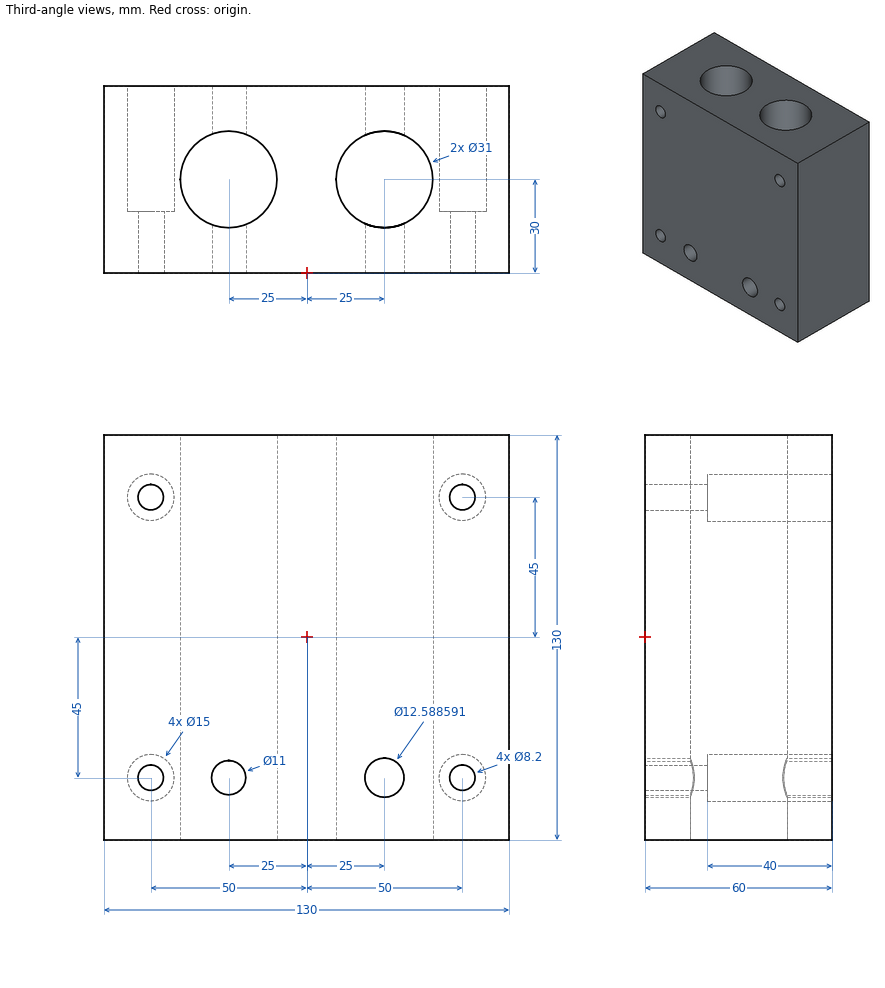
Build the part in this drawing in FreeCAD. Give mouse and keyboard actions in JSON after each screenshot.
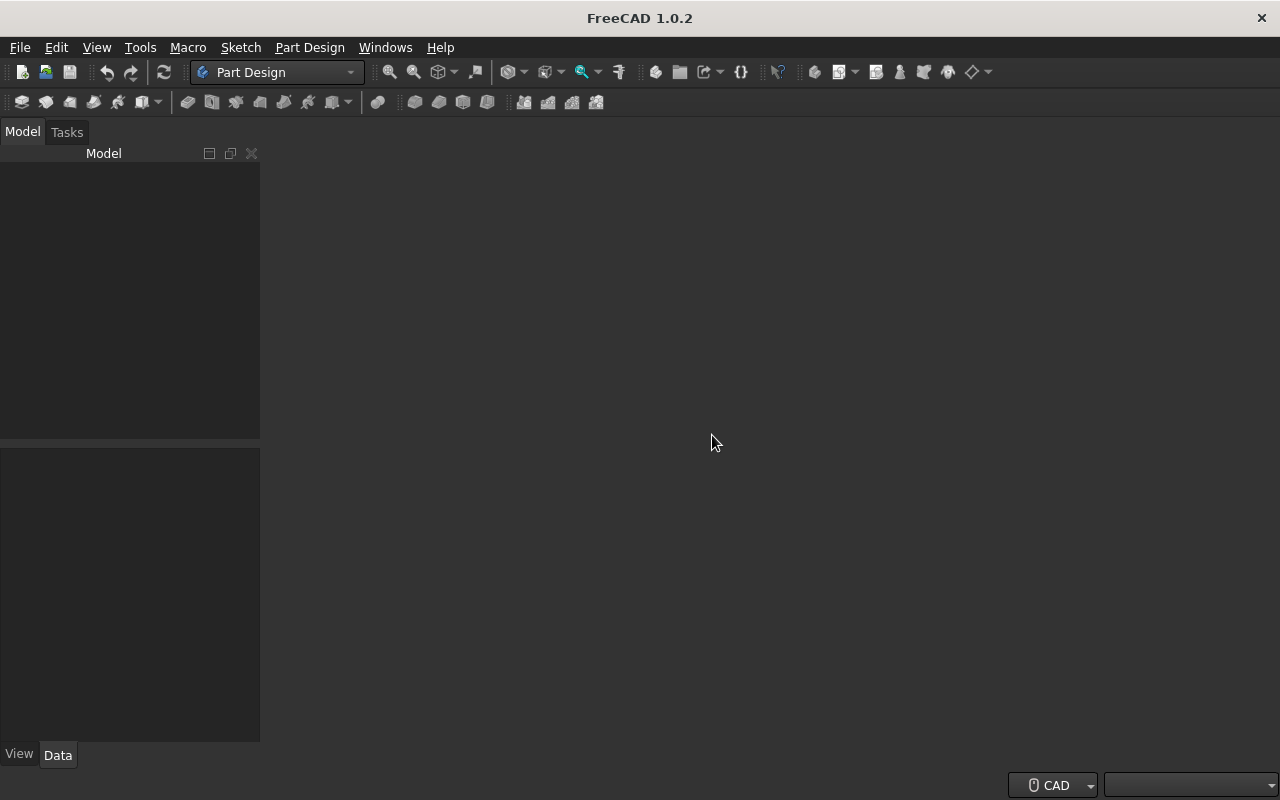
{"action": "key", "text": "ctrl+n"}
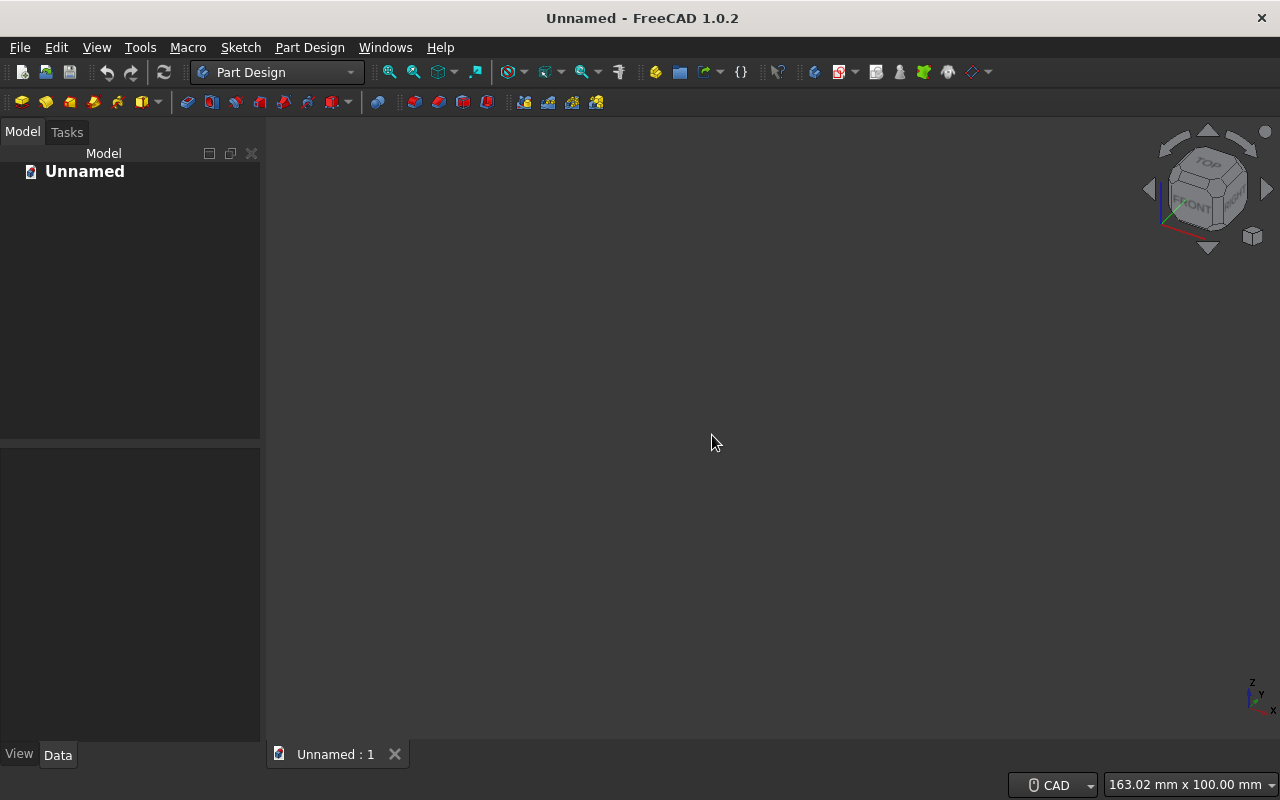
{"action": "left_click", "coordinate": [840, 72]}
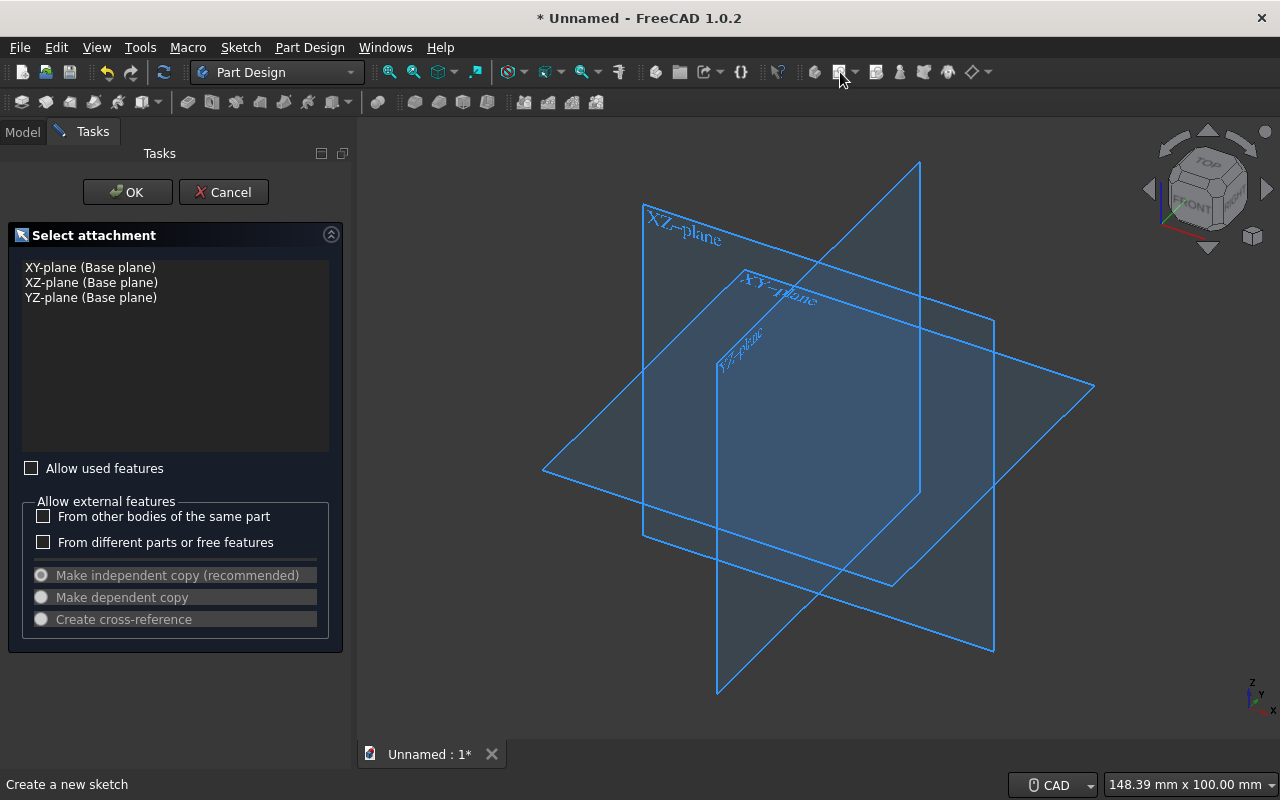
{"action": "left_click", "coordinate": [82, 282]}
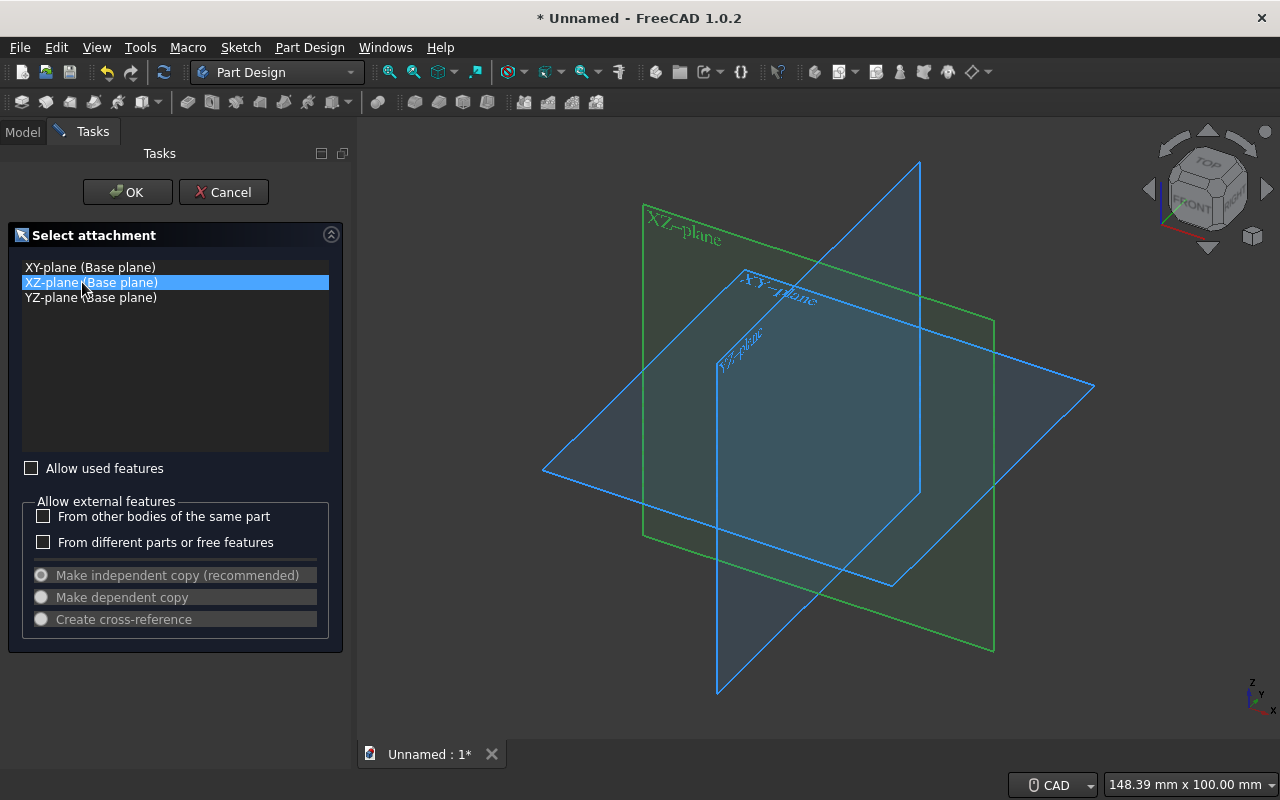
{"action": "left_click", "coordinate": [128, 192]}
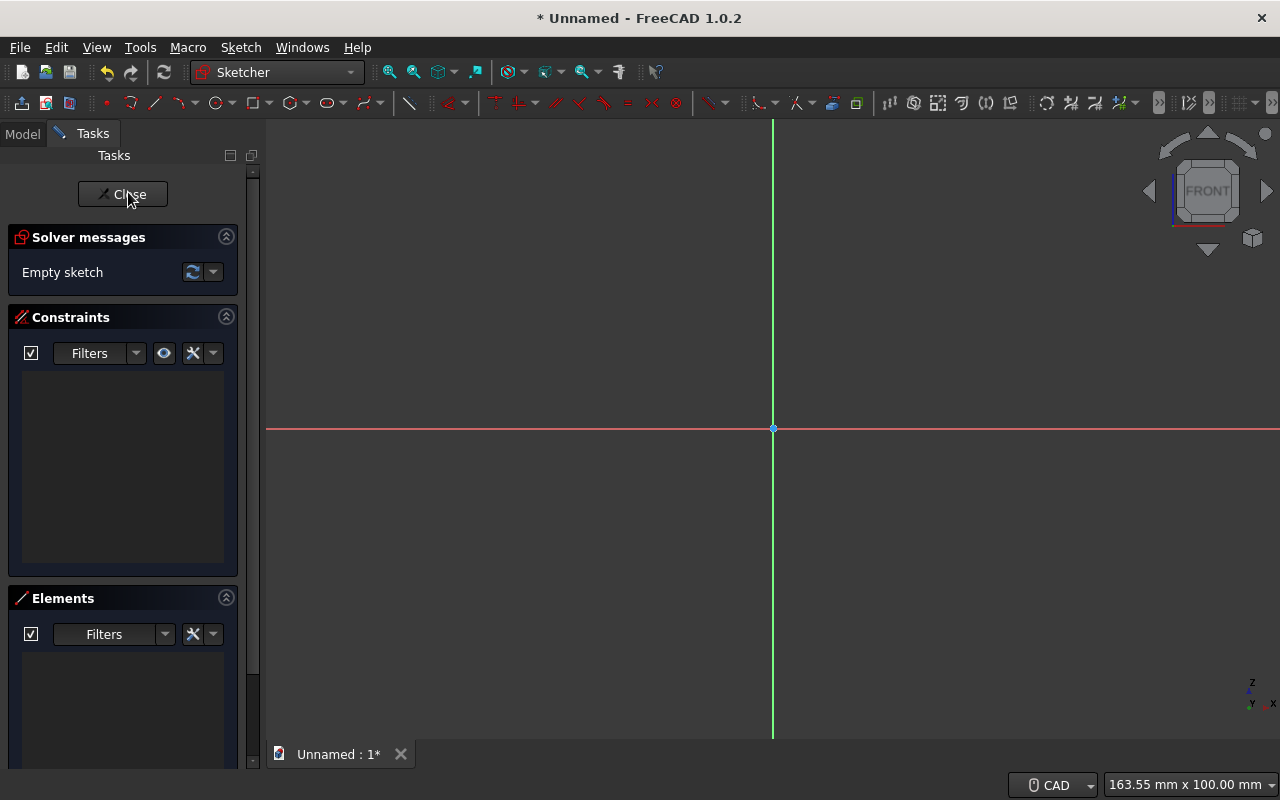
{"action": "scroll", "coordinate": [649, 429], "scroll_direction": "down", "scroll_amount": 4}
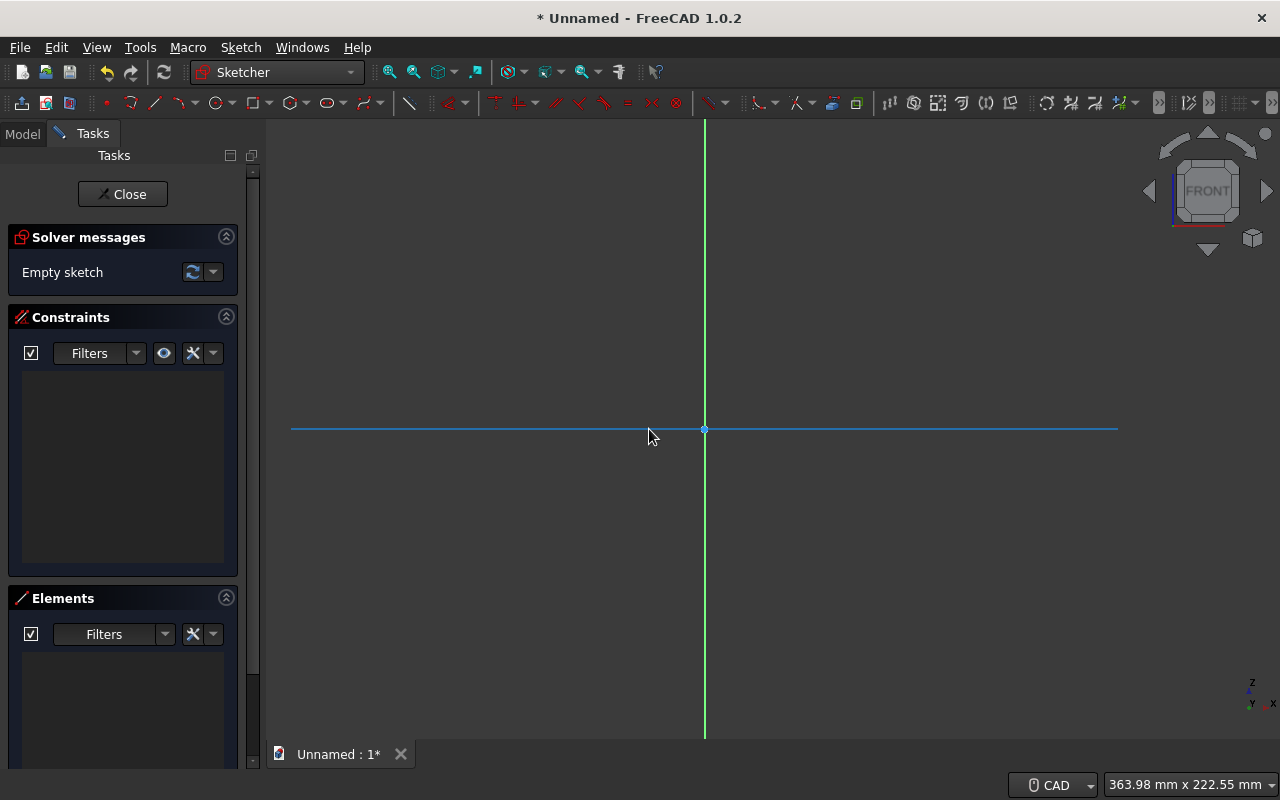
{"action": "key", "text": "g v"}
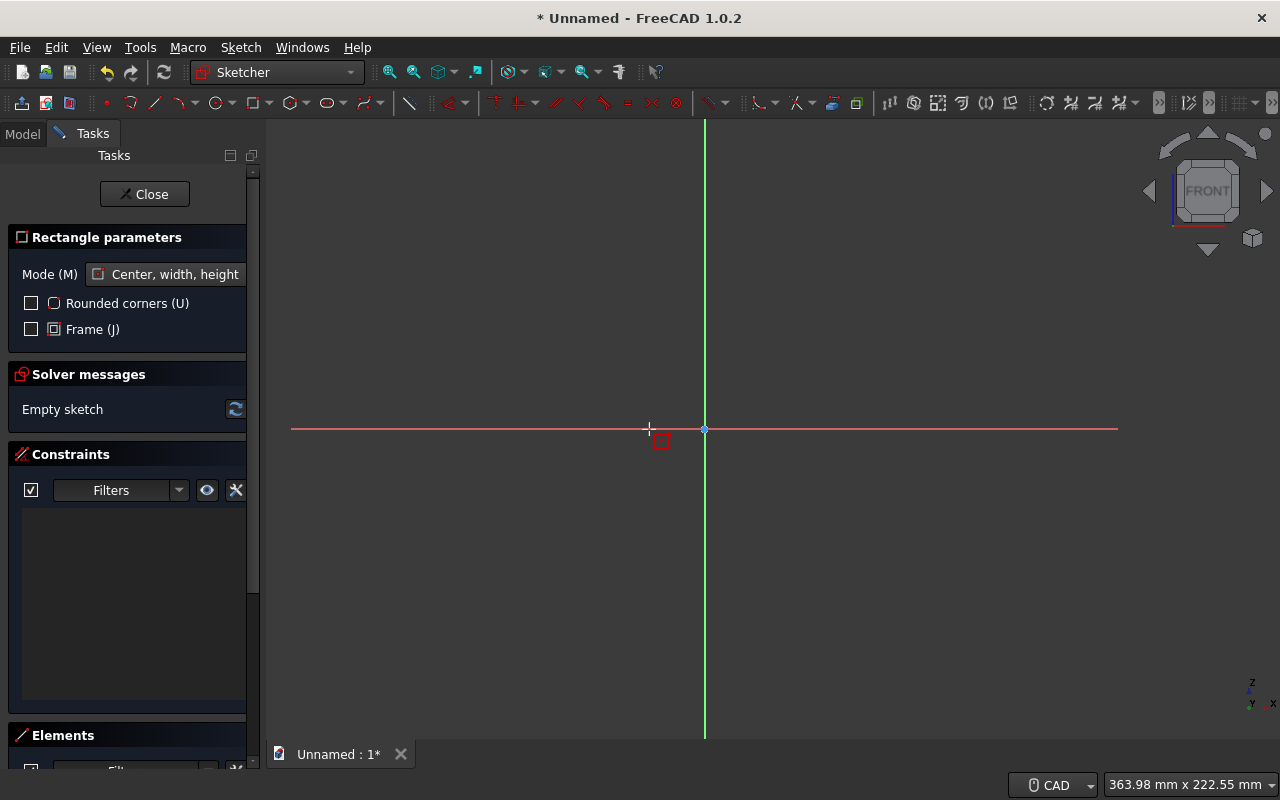
{"action": "left_click", "coordinate": [705, 429]}
{"action": "left_click", "coordinate": [886, 248]}
{"action": "key", "text": "Escape"}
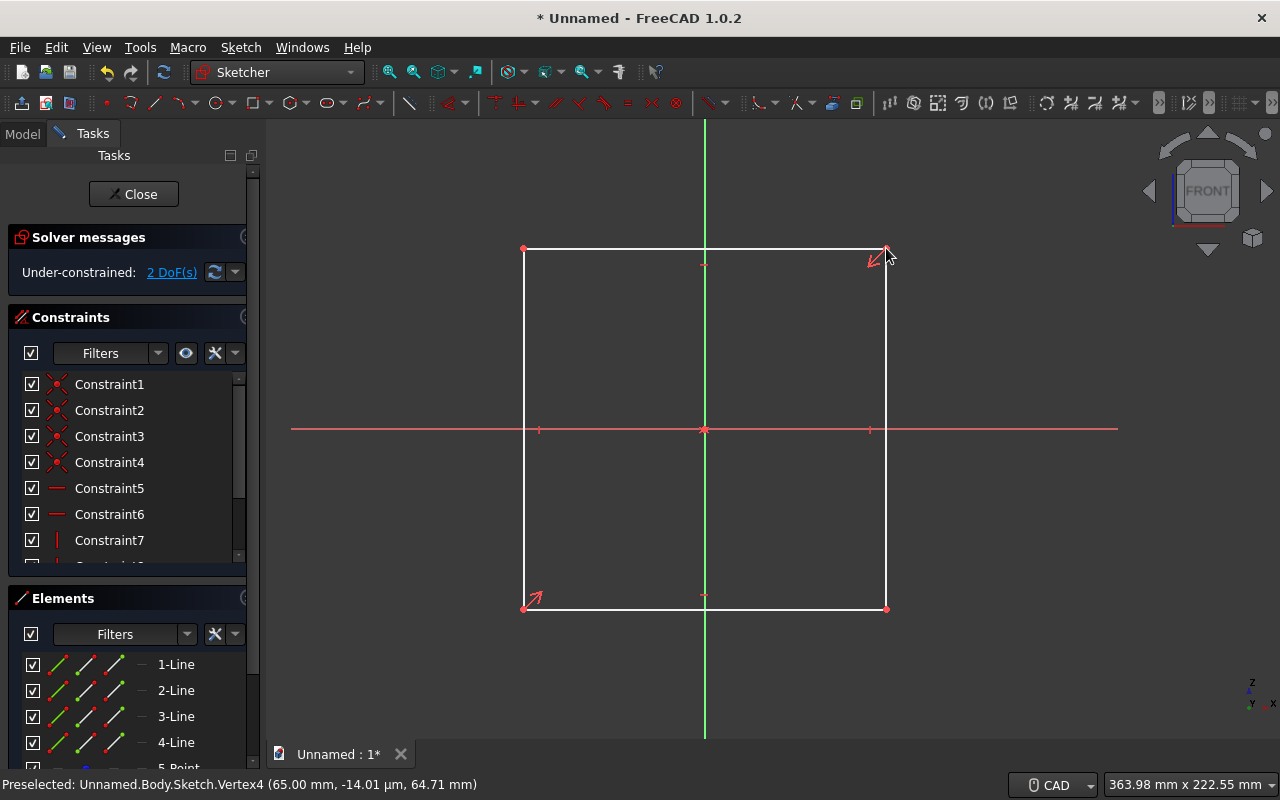
{"action": "left_click", "coordinate": [632, 610]}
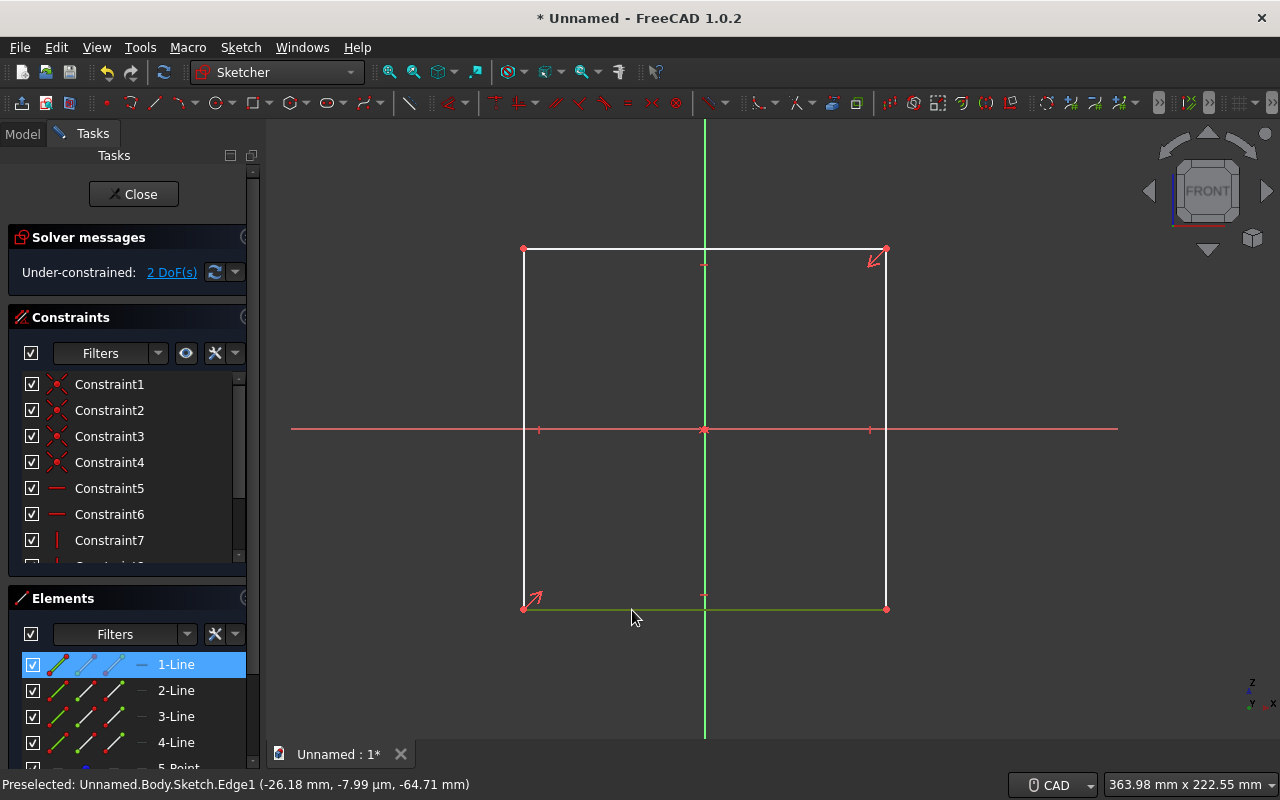
{"action": "key", "text": "l"}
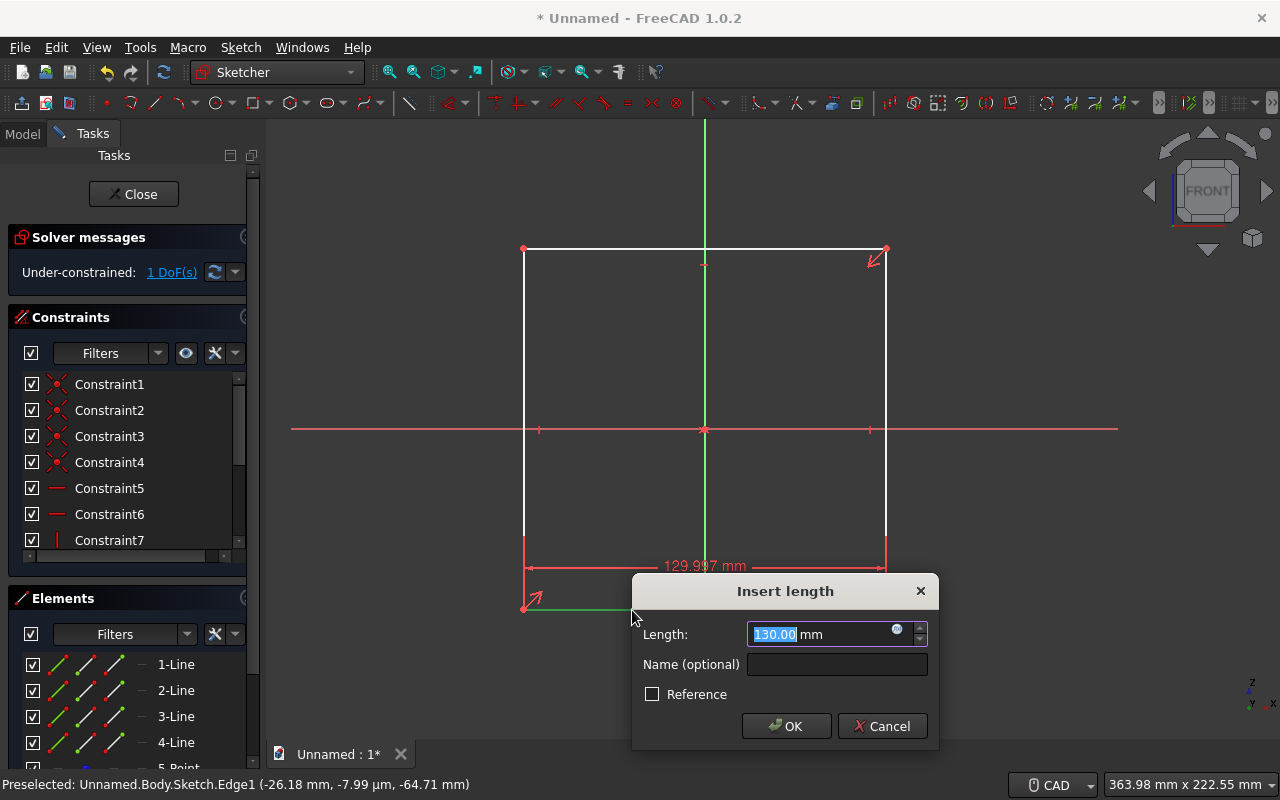
{"action": "type", "text": "130"}
{"action": "key", "text": "Return"}